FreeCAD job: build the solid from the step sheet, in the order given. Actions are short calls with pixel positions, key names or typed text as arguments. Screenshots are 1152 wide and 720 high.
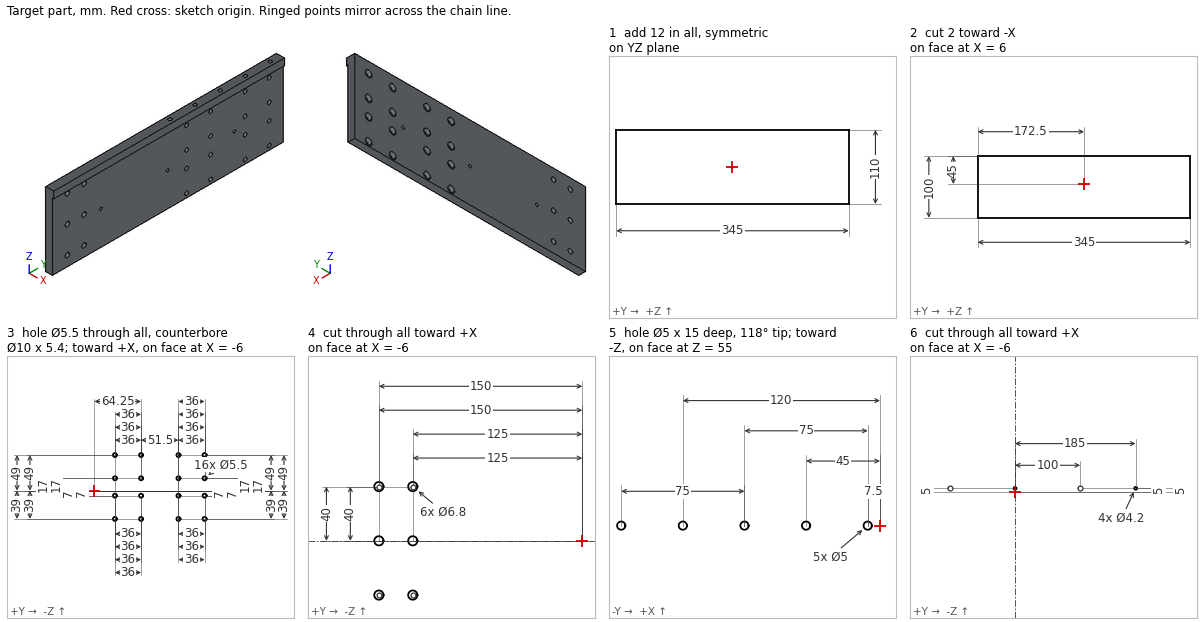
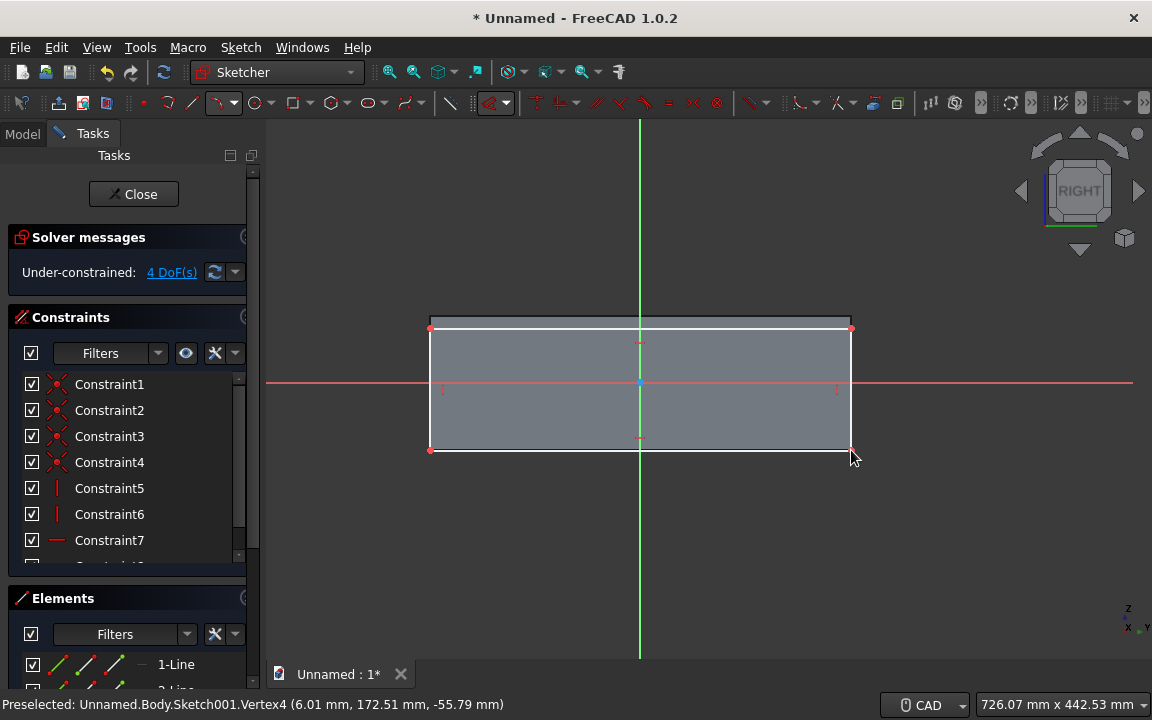
click(430, 366)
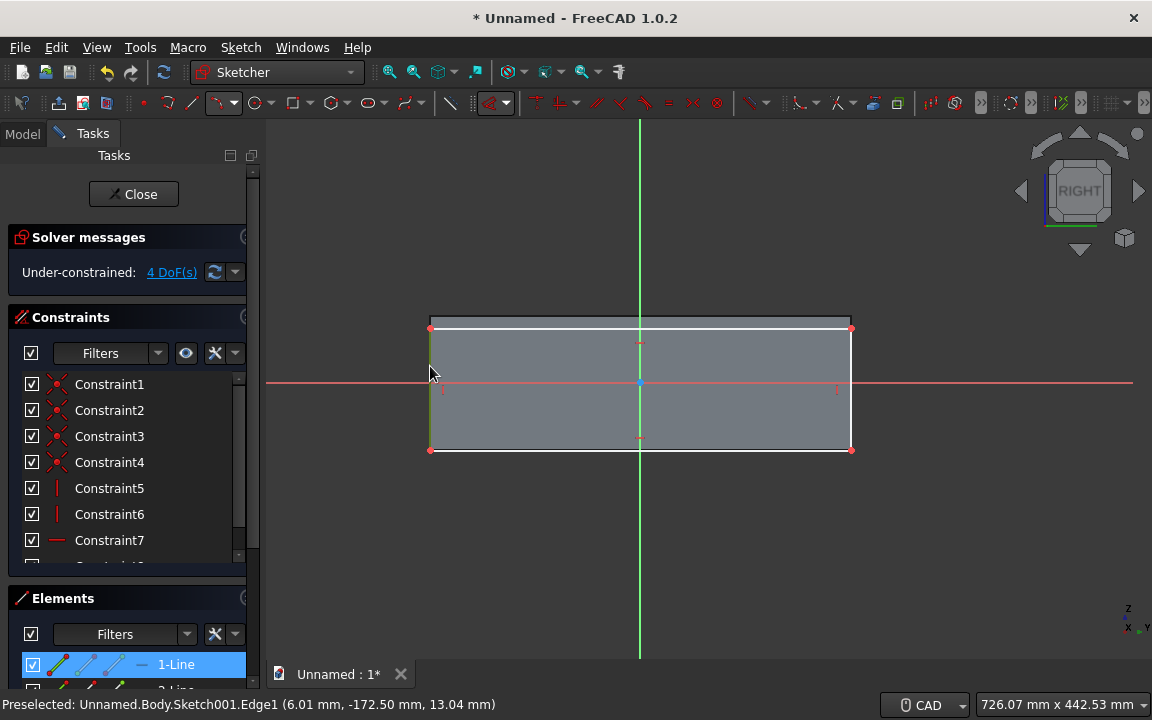
click(508, 104)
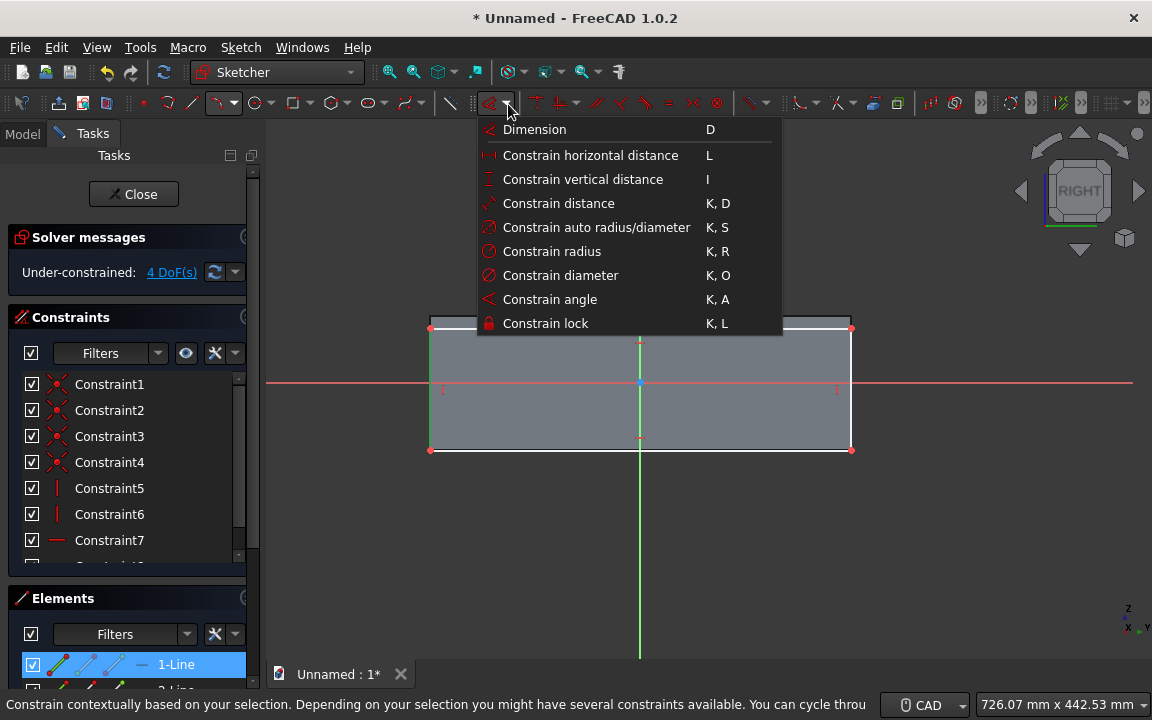
click(630, 179)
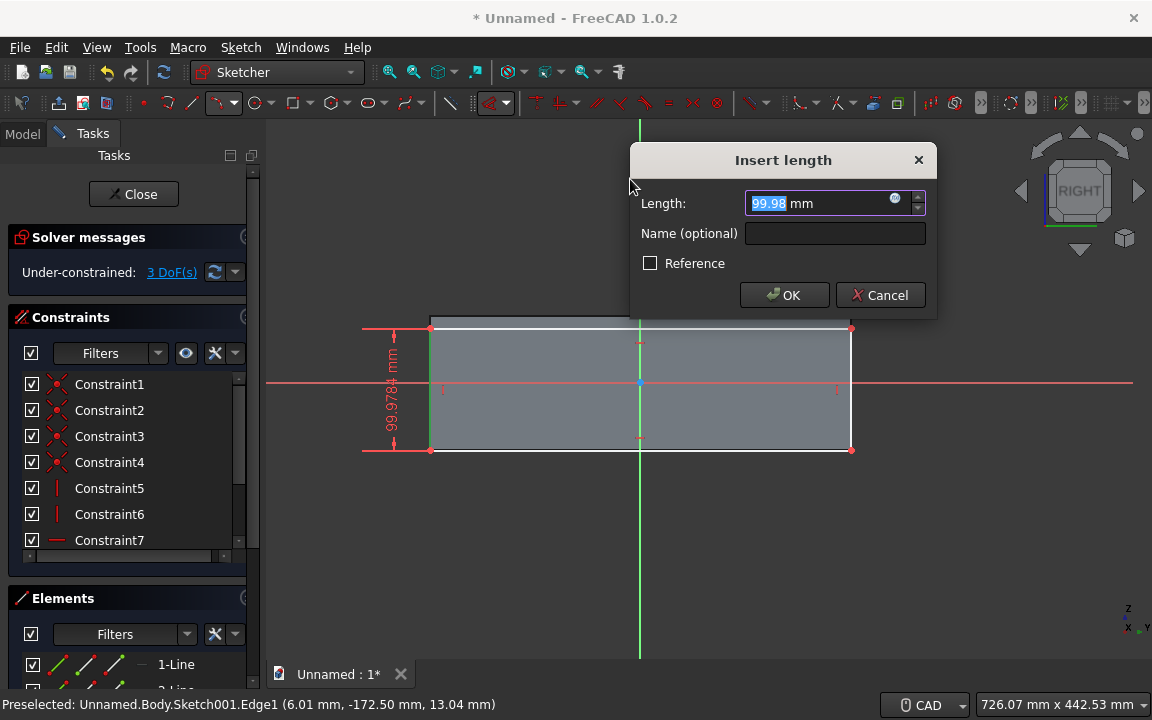
text(100)
key(Return)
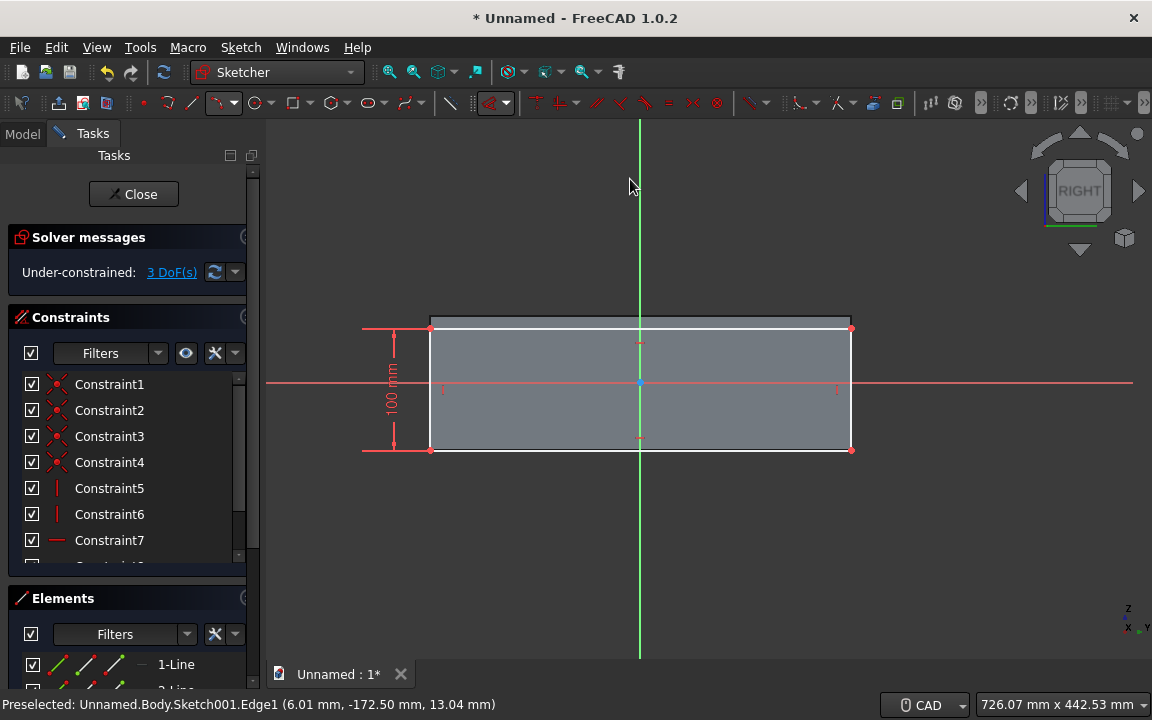
click(556, 451)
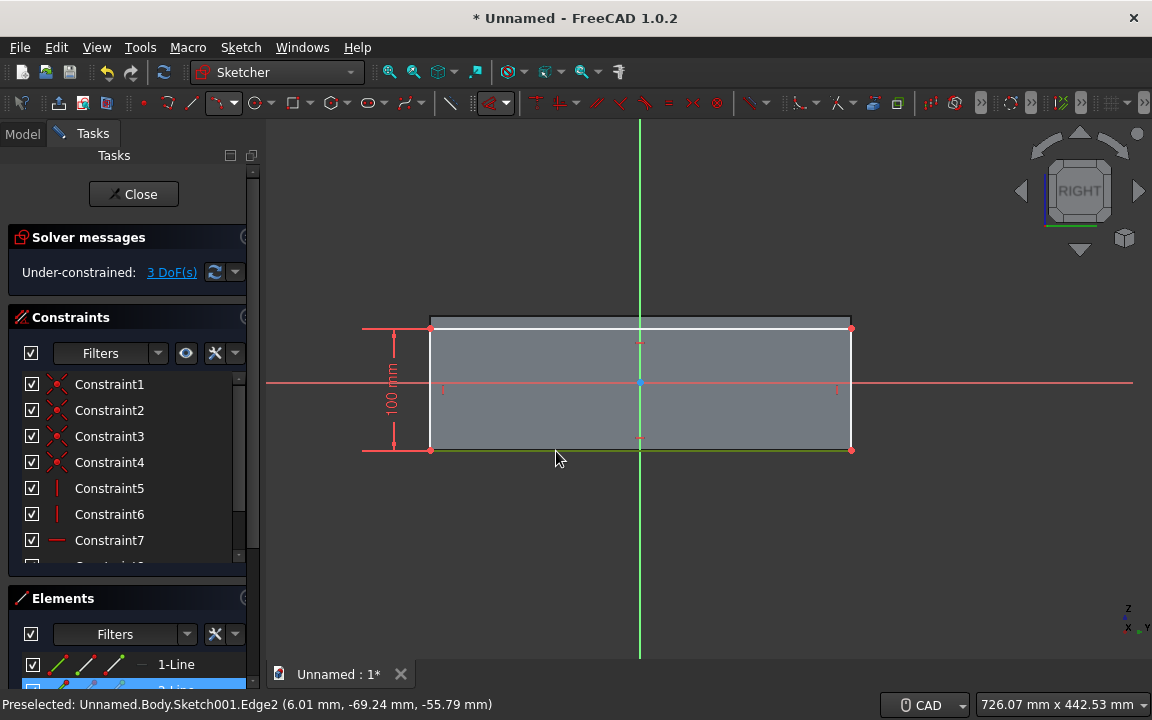
key(l)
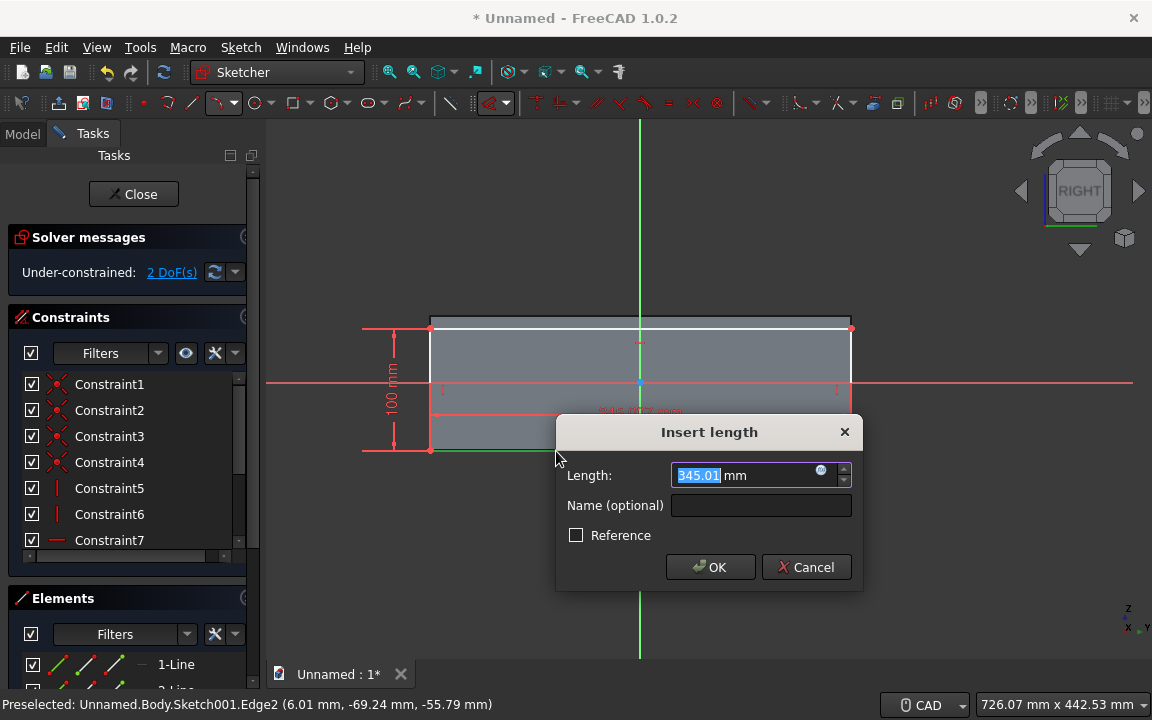
text(345)
key(Return)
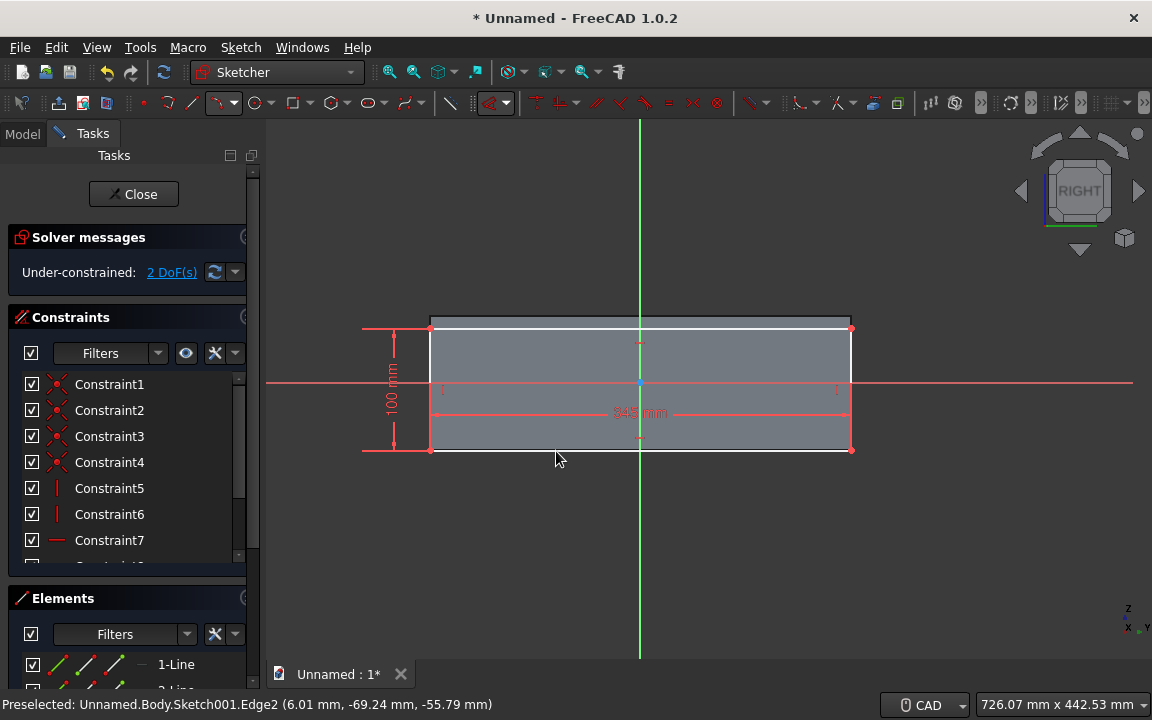
click(430, 329)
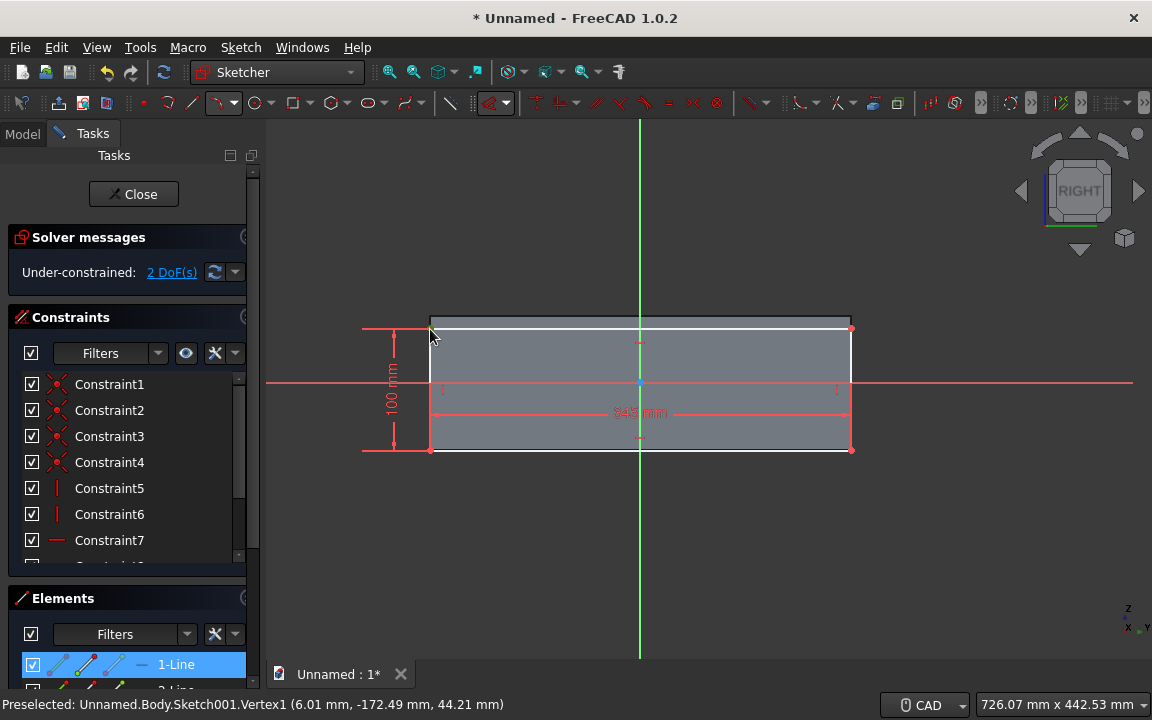
click(508, 104)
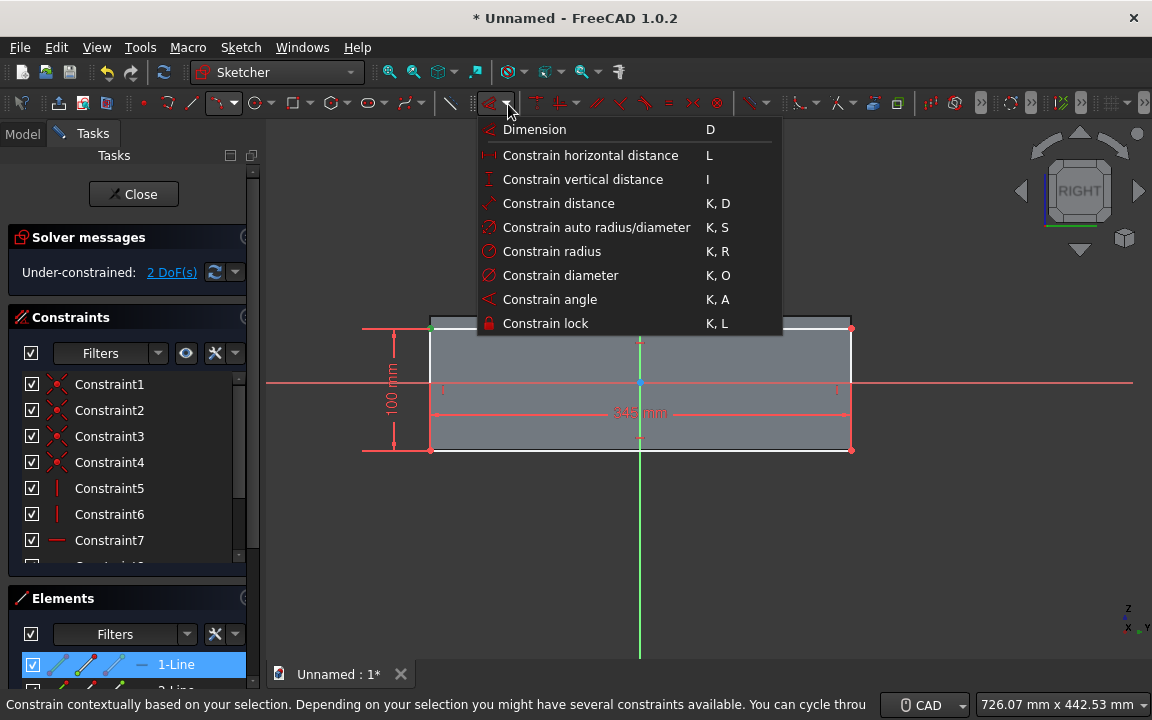
click(630, 179)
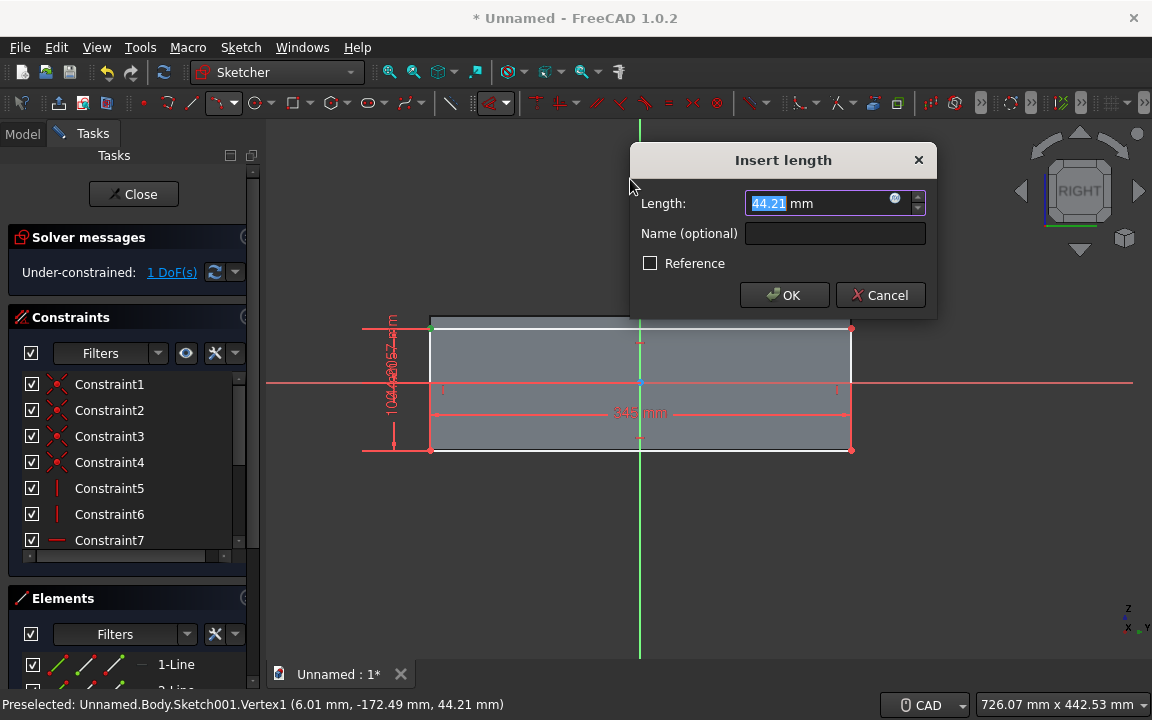
text(45)
key(Return)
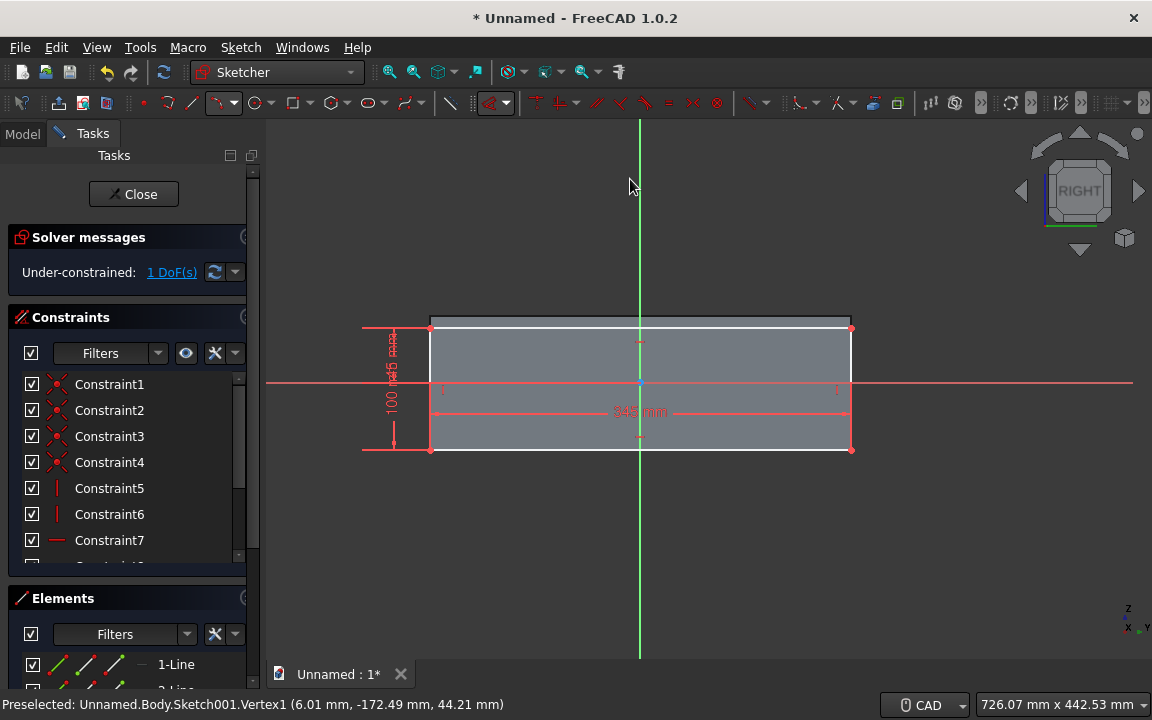
click(430, 328)